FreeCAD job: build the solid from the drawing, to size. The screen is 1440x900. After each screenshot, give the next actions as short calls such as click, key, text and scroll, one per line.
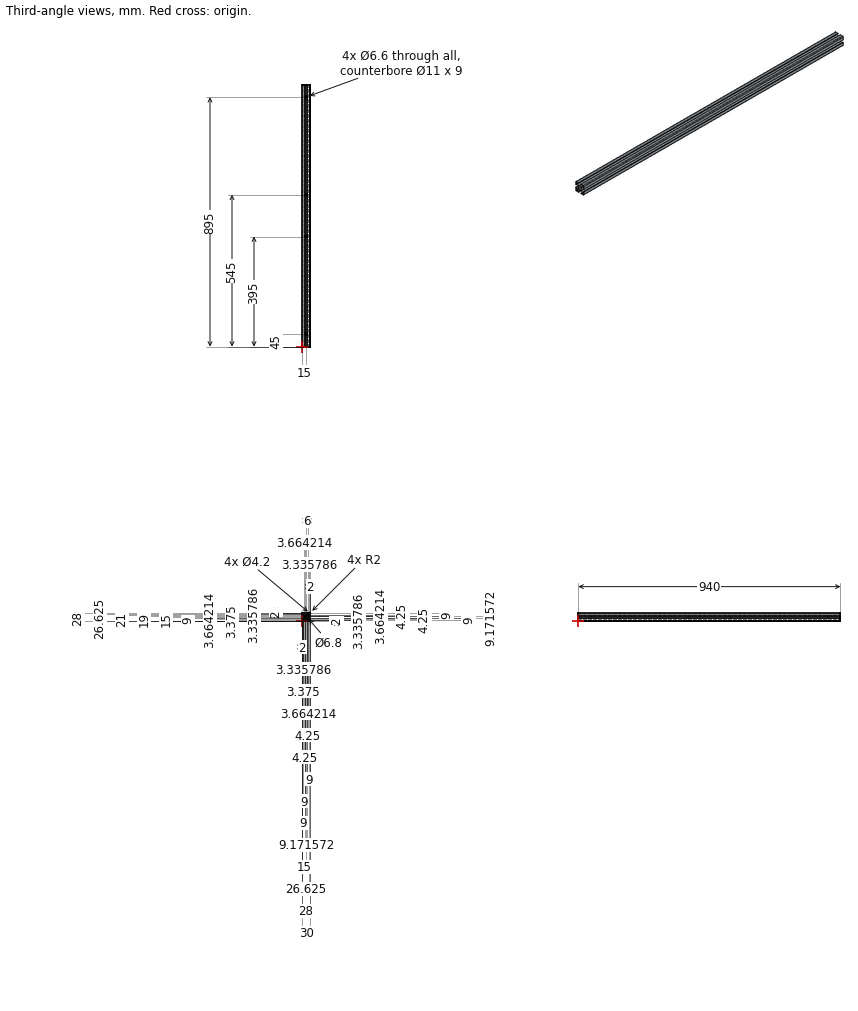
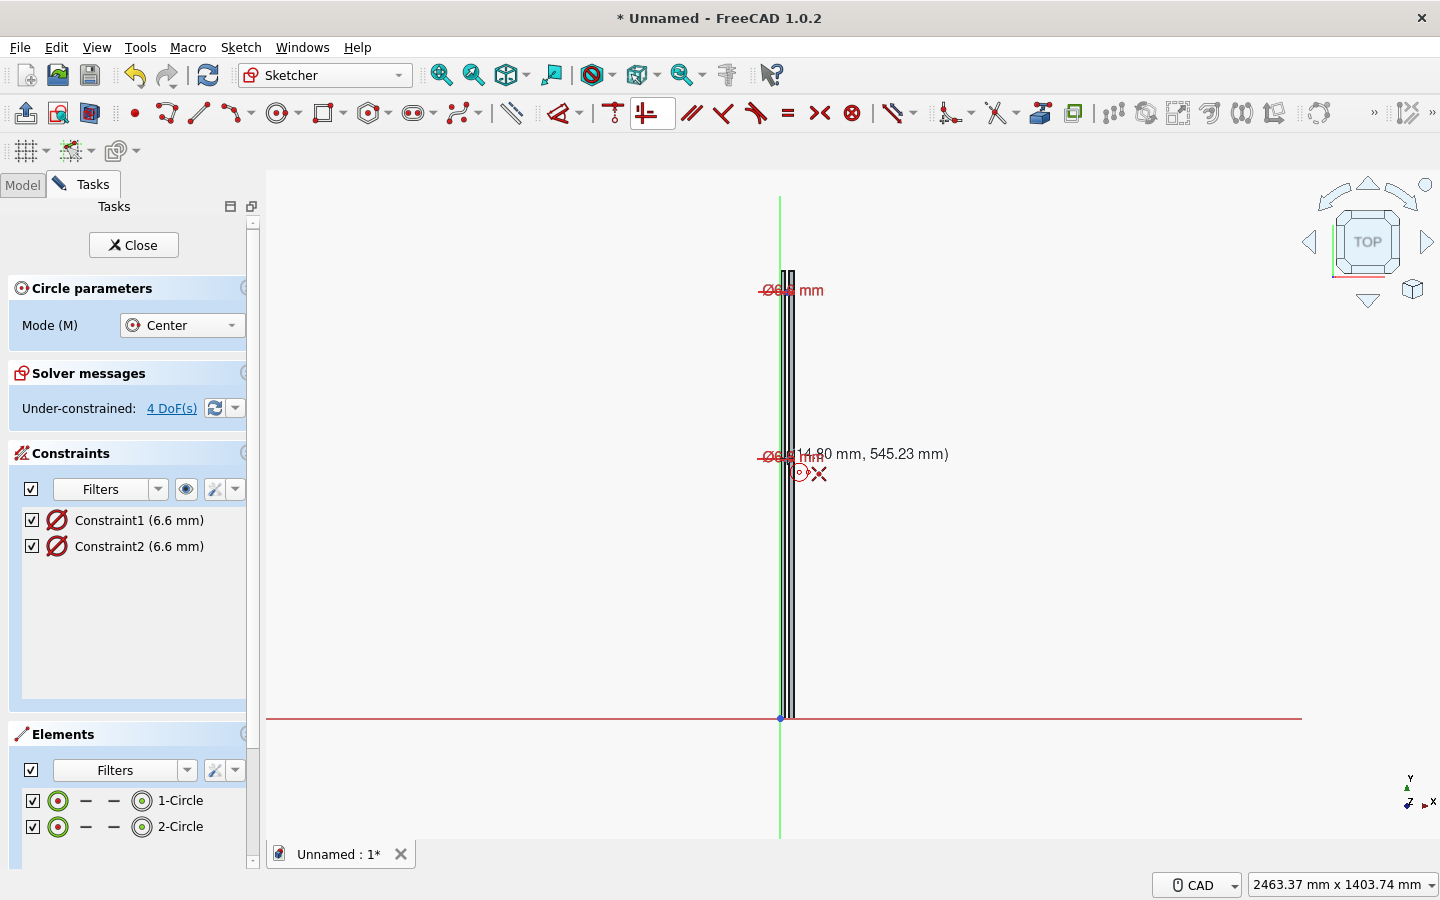
scroll(787, 697, up, 14)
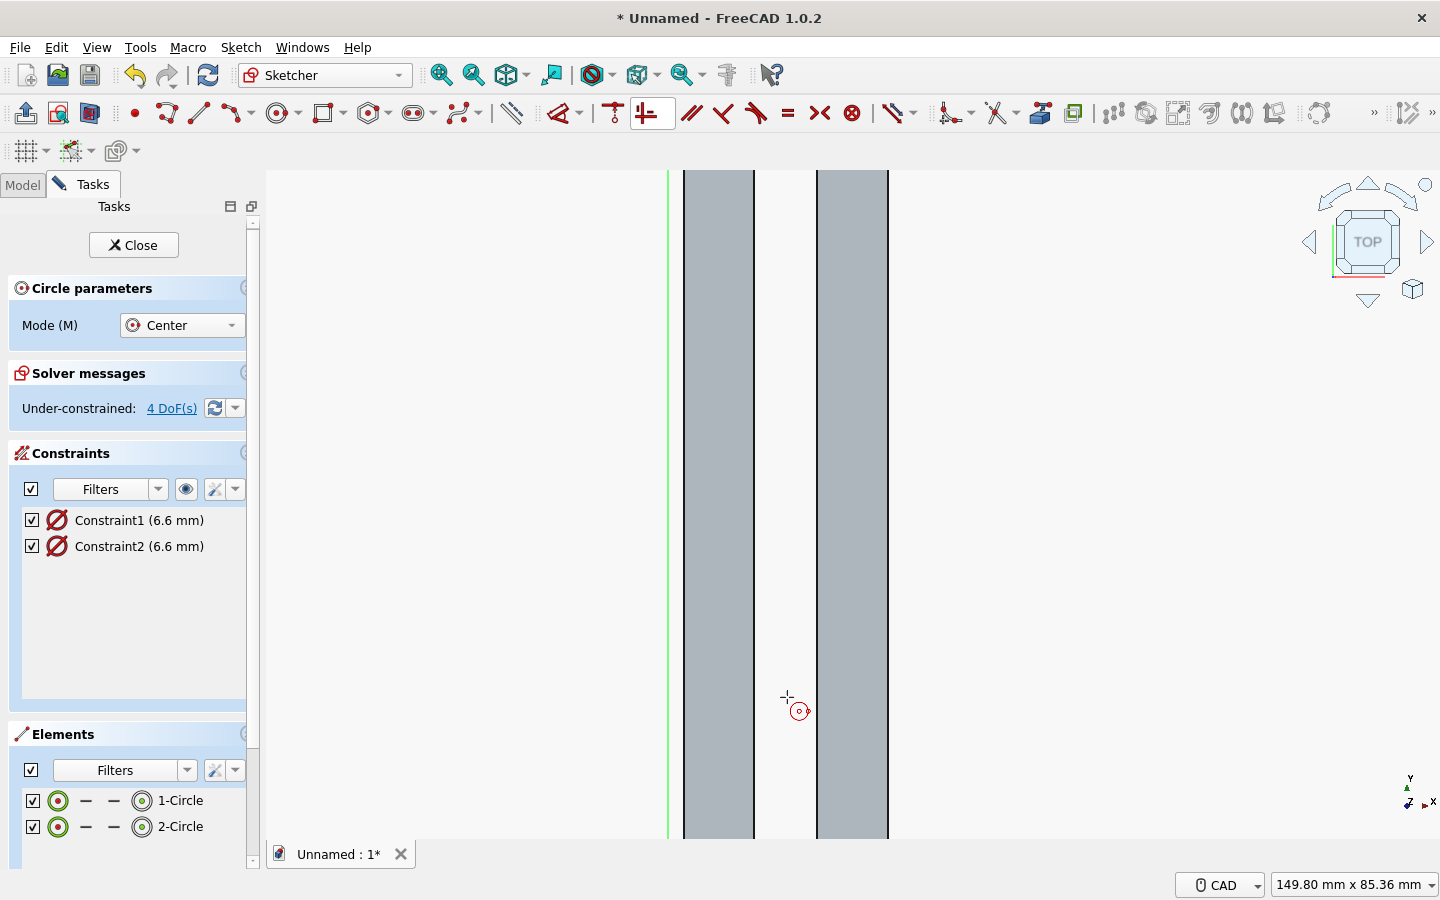
scroll(787, 698, down, 14)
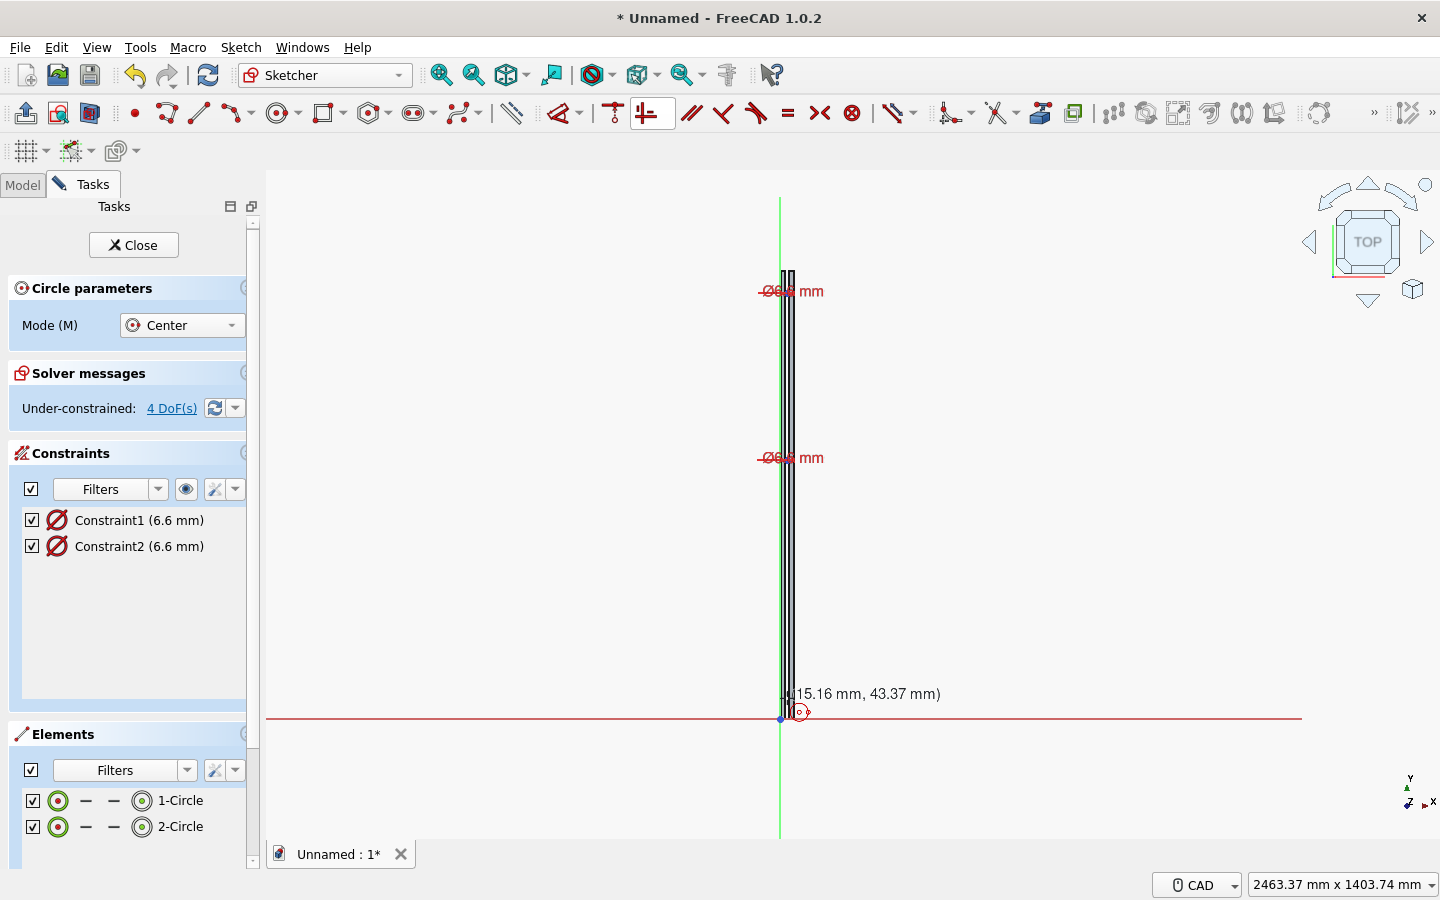
scroll(787, 698, up, 4)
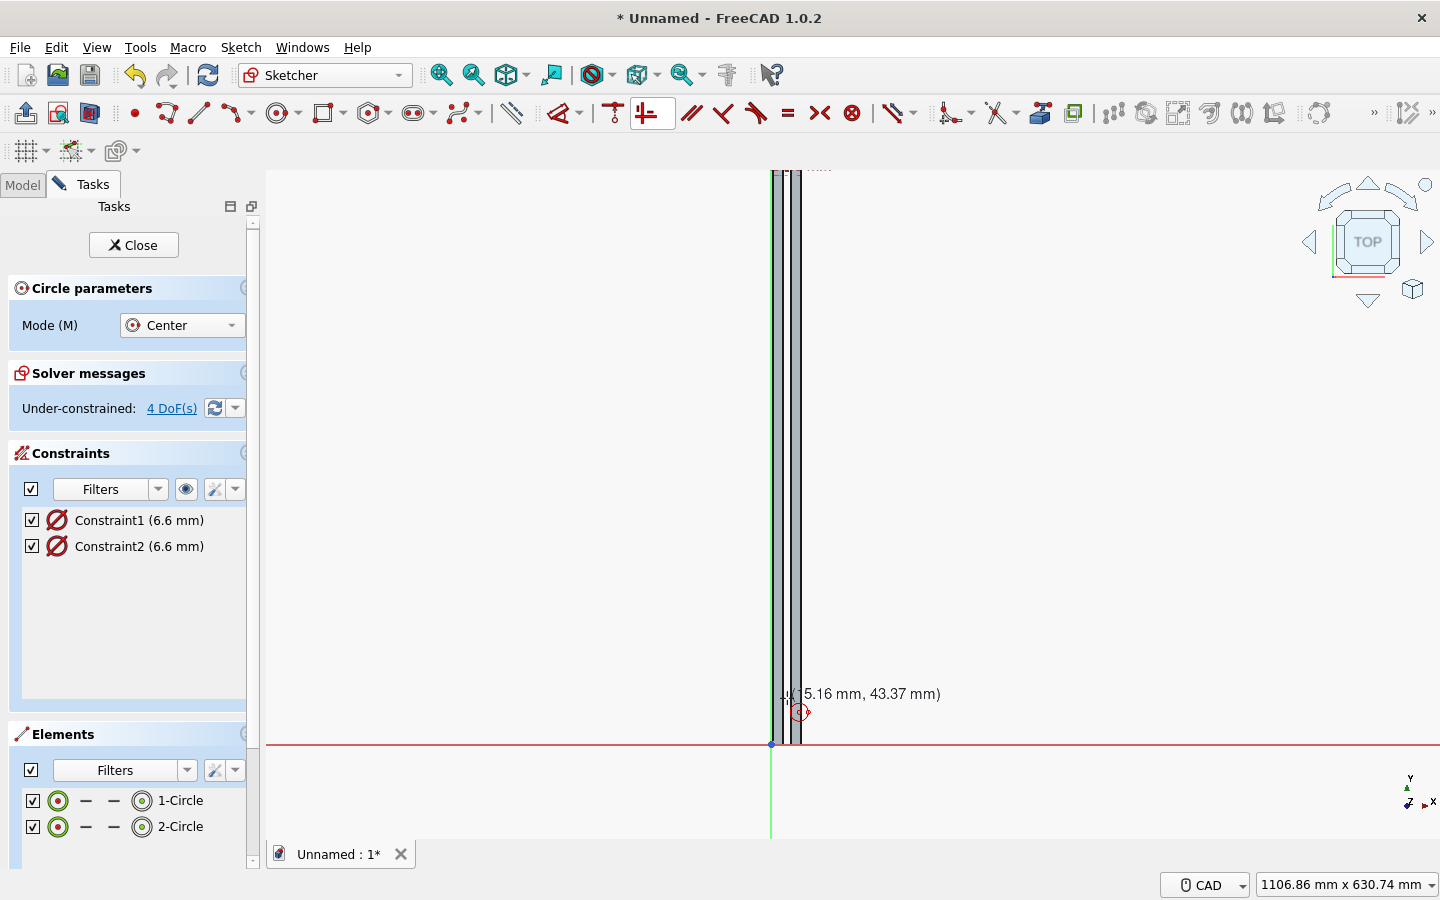
click(787, 697)
move(790, 695)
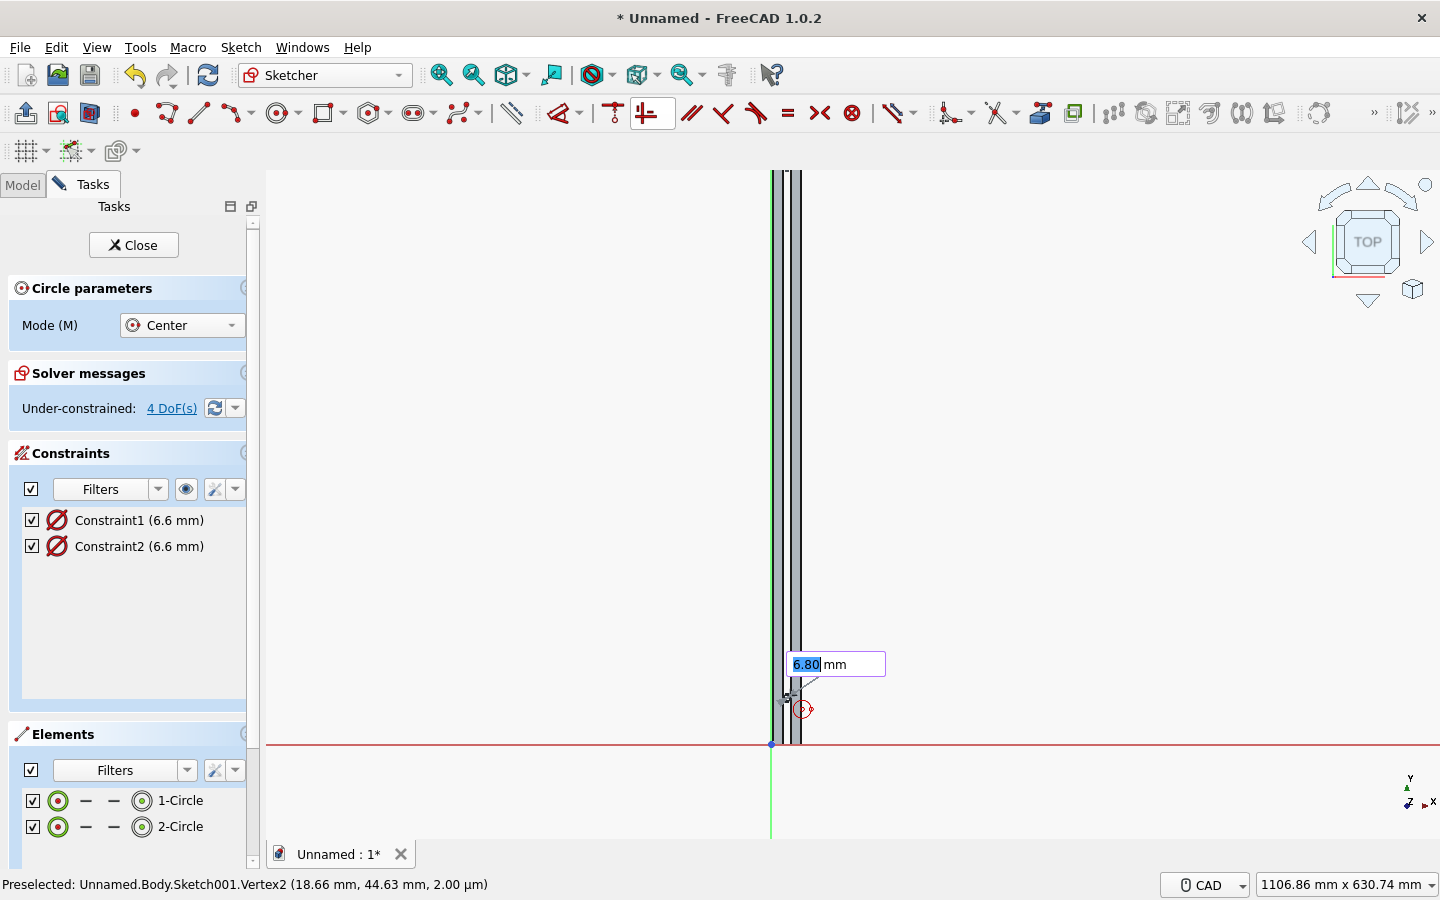
text(6.6)
key(Return)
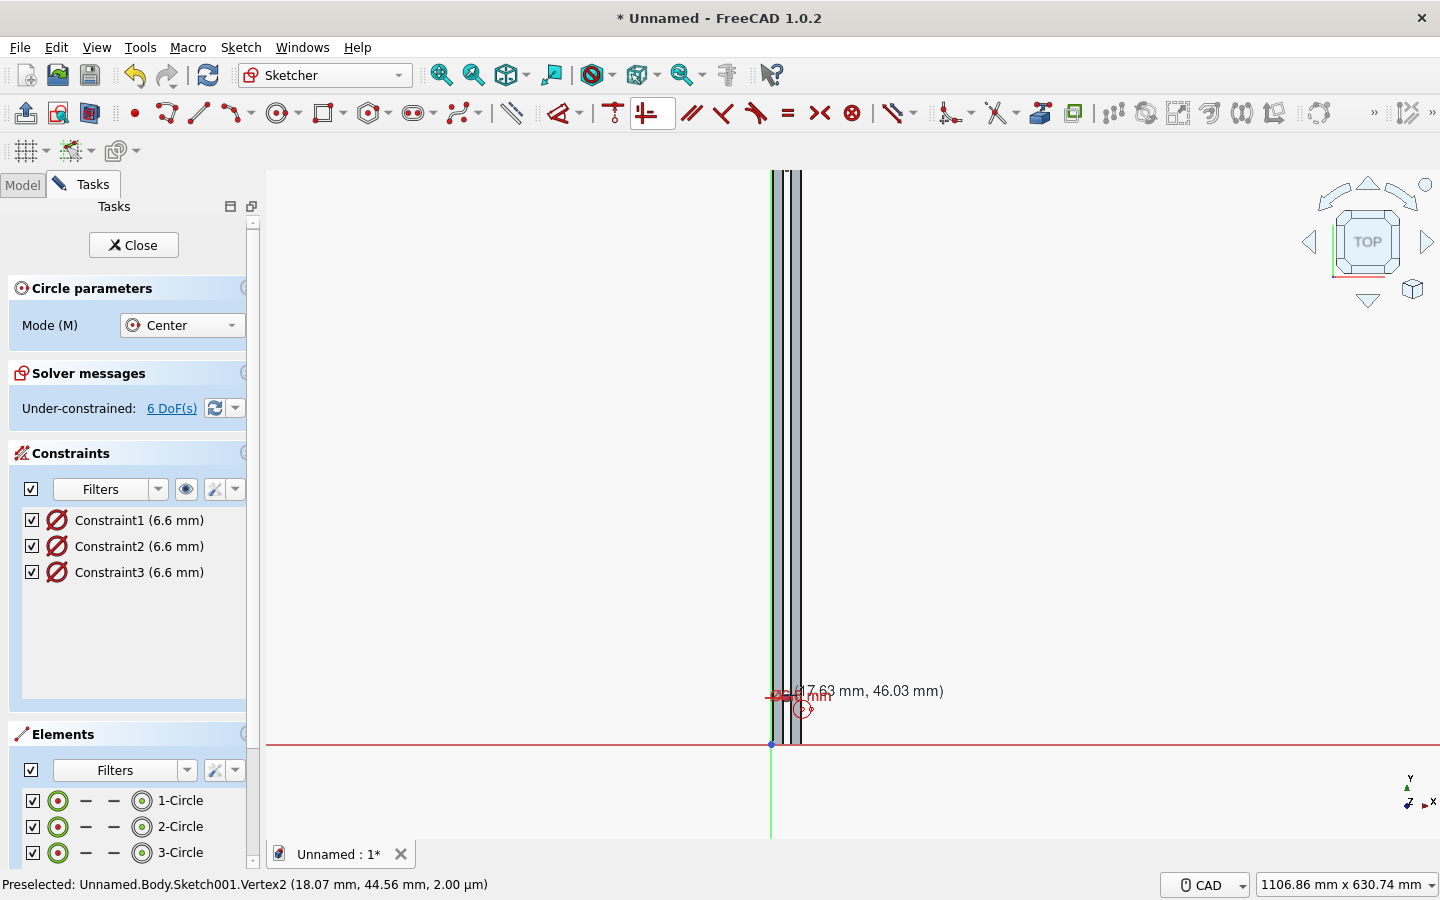
scroll(787, 326, up, 10)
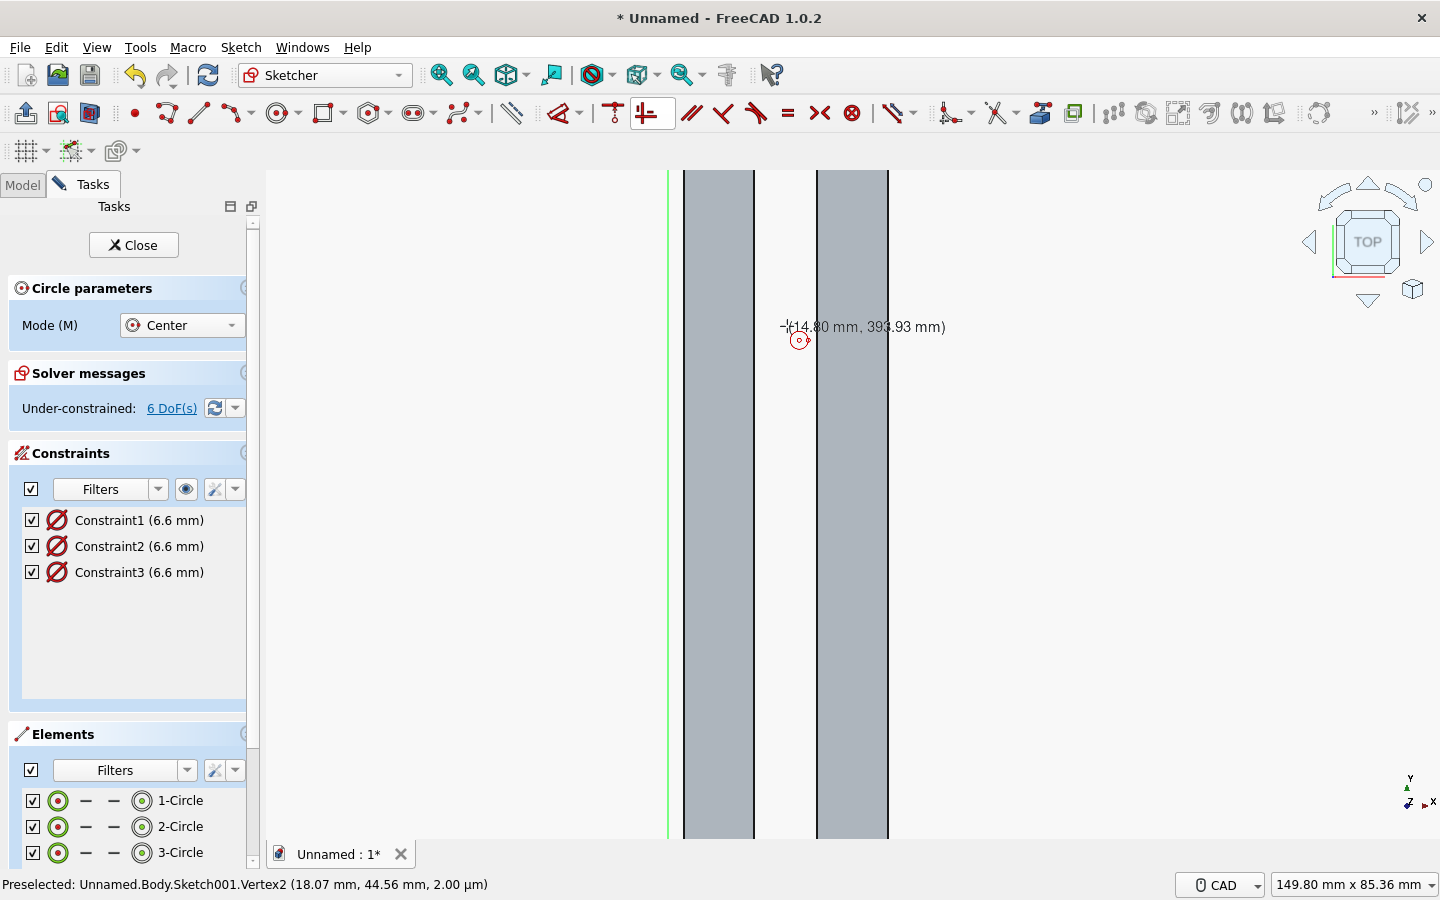
scroll(787, 544, down, 14)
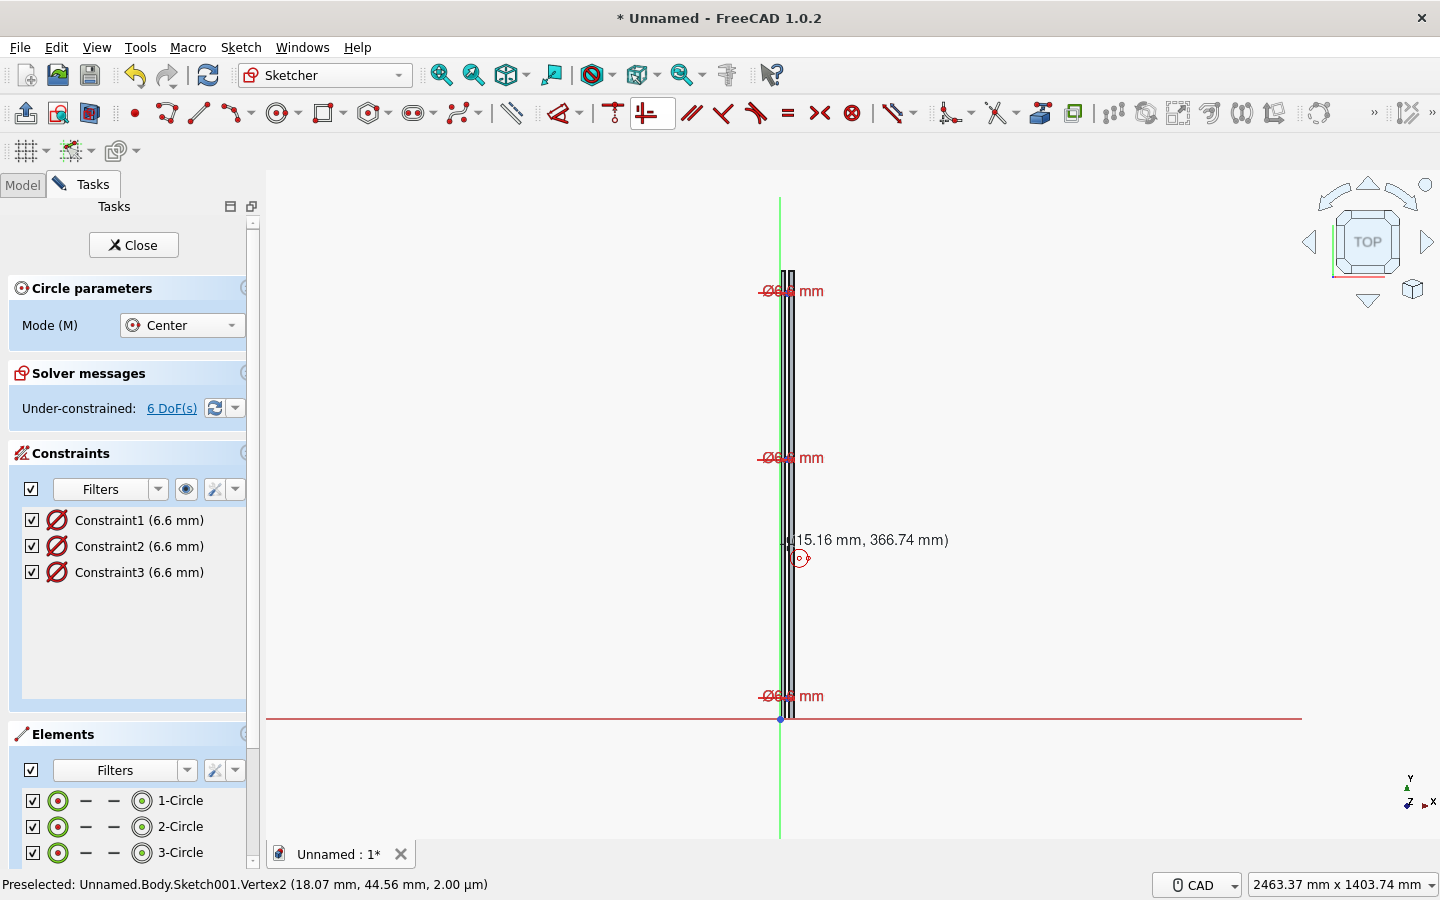
scroll(787, 531, up, 4)